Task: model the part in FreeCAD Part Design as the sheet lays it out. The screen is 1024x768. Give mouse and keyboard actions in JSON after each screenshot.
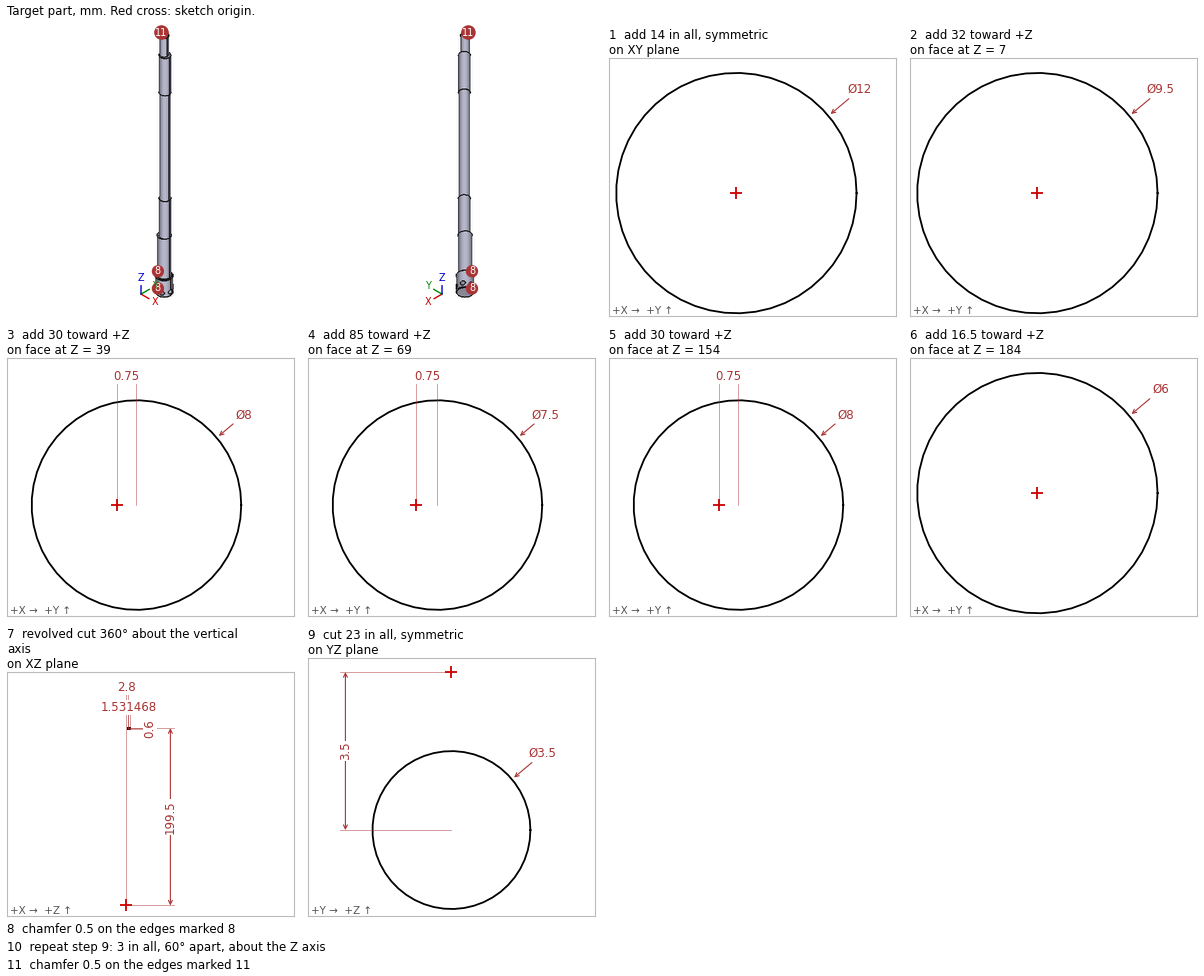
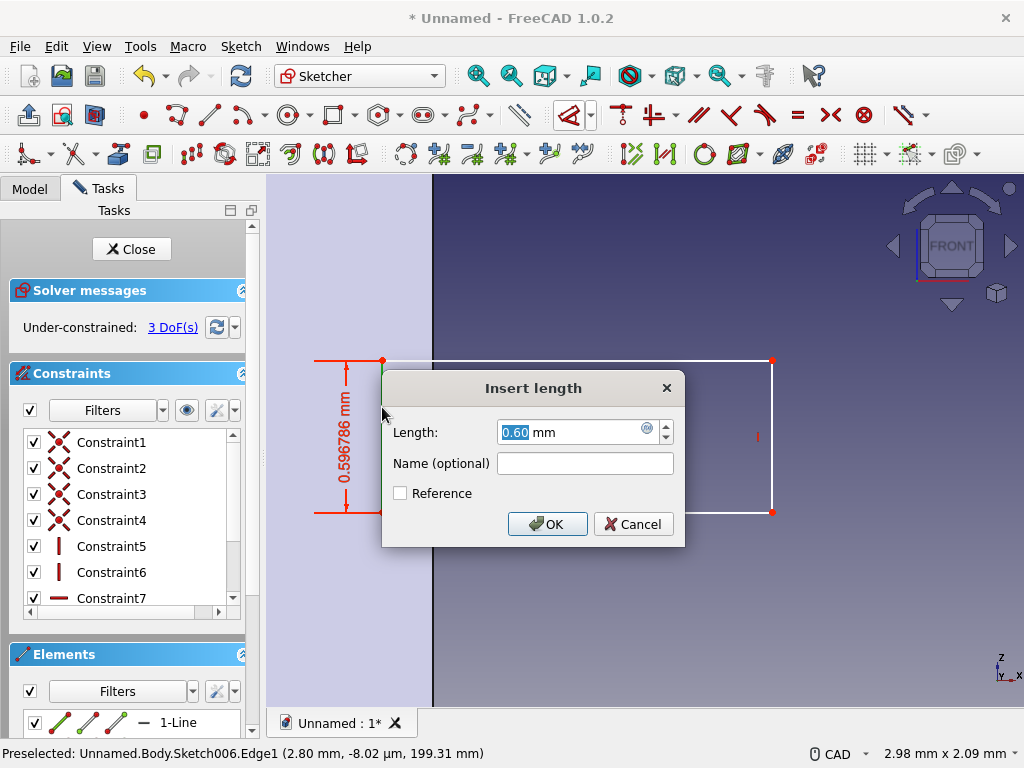
{"action": "type", "text": "0.6"}
{"action": "key", "text": "Return"}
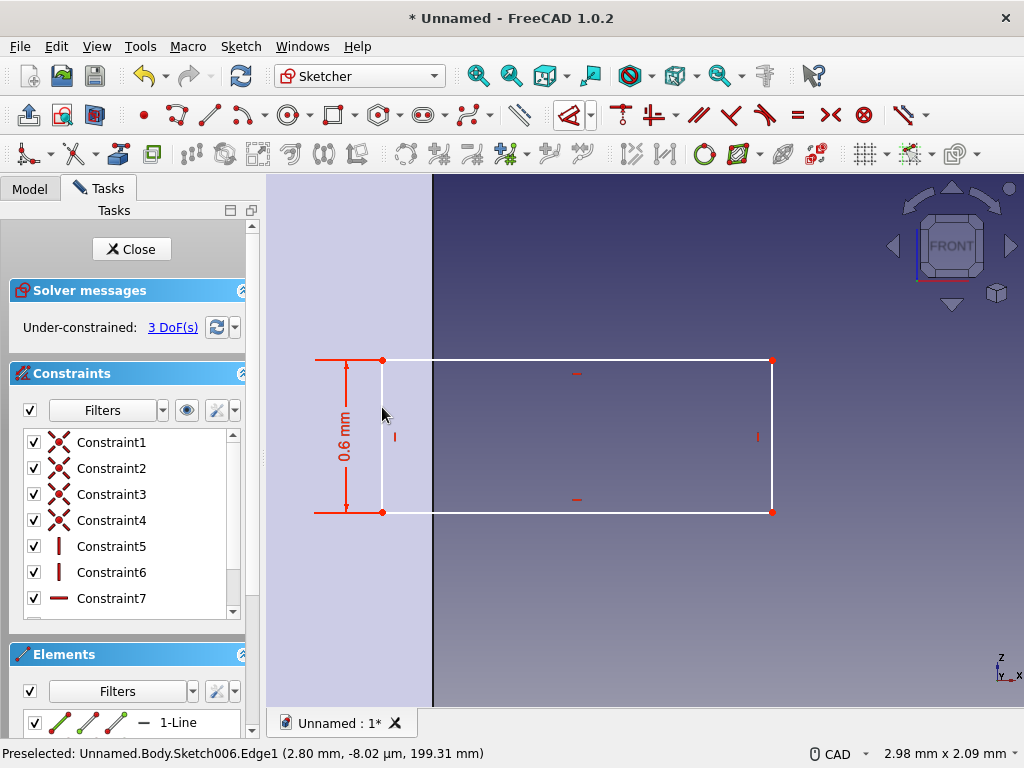
{"action": "left_click", "coordinate": [382, 360]}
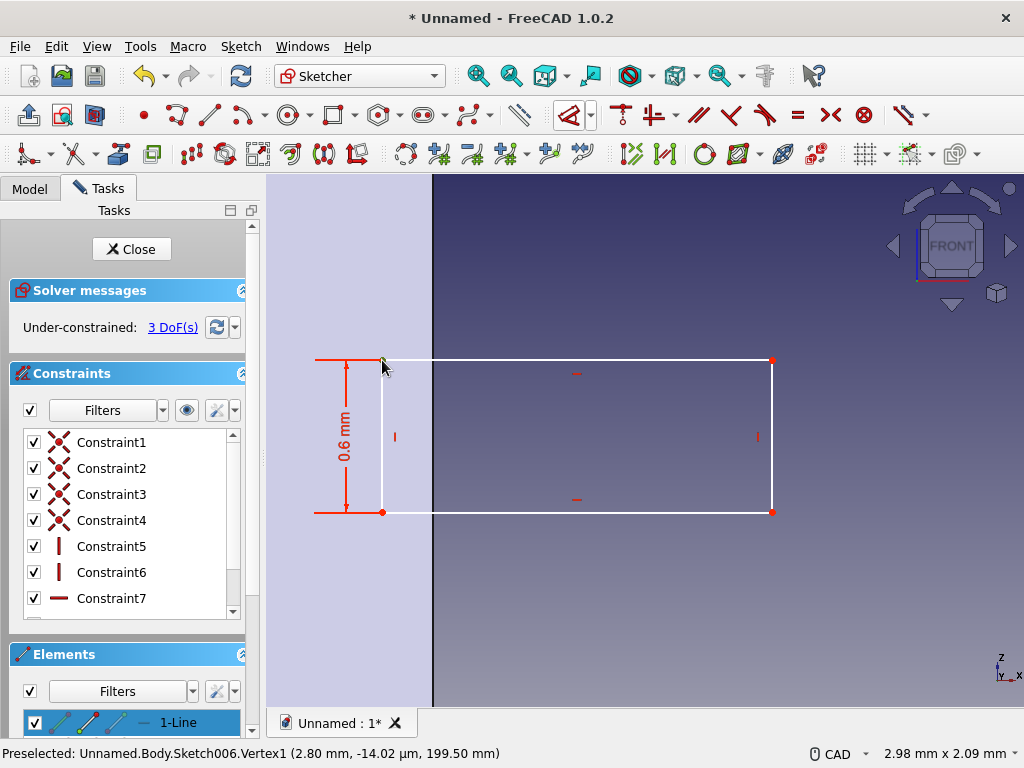
{"action": "key", "text": "l"}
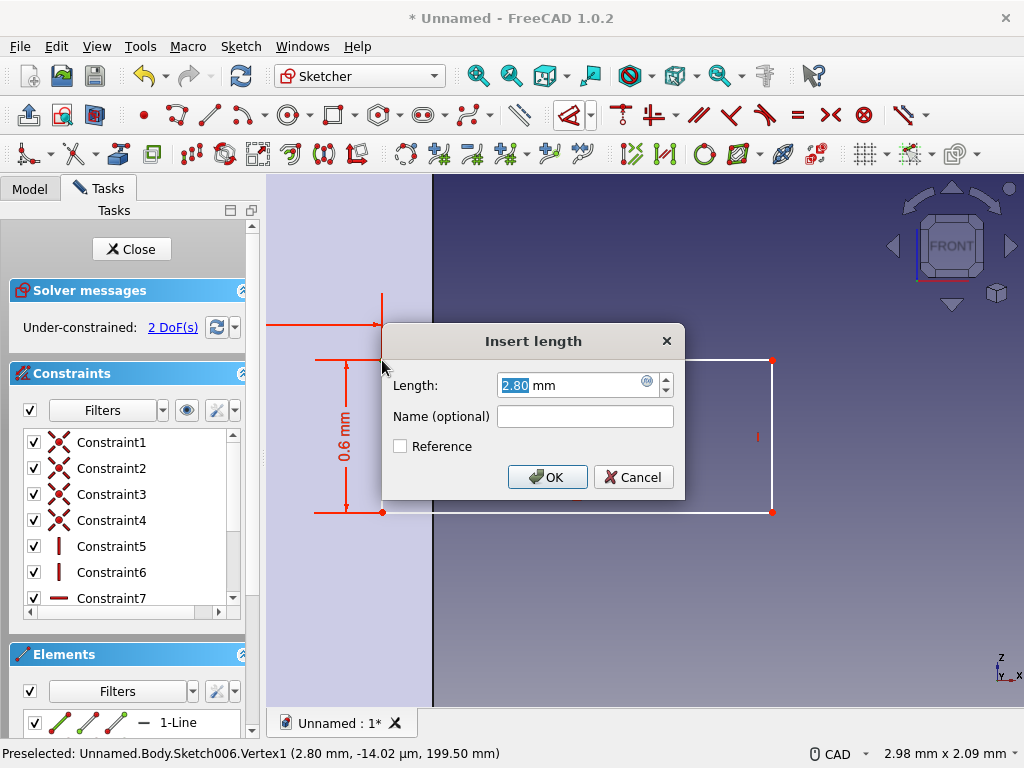
{"action": "type", "text": "2.8"}
{"action": "key", "text": "Return"}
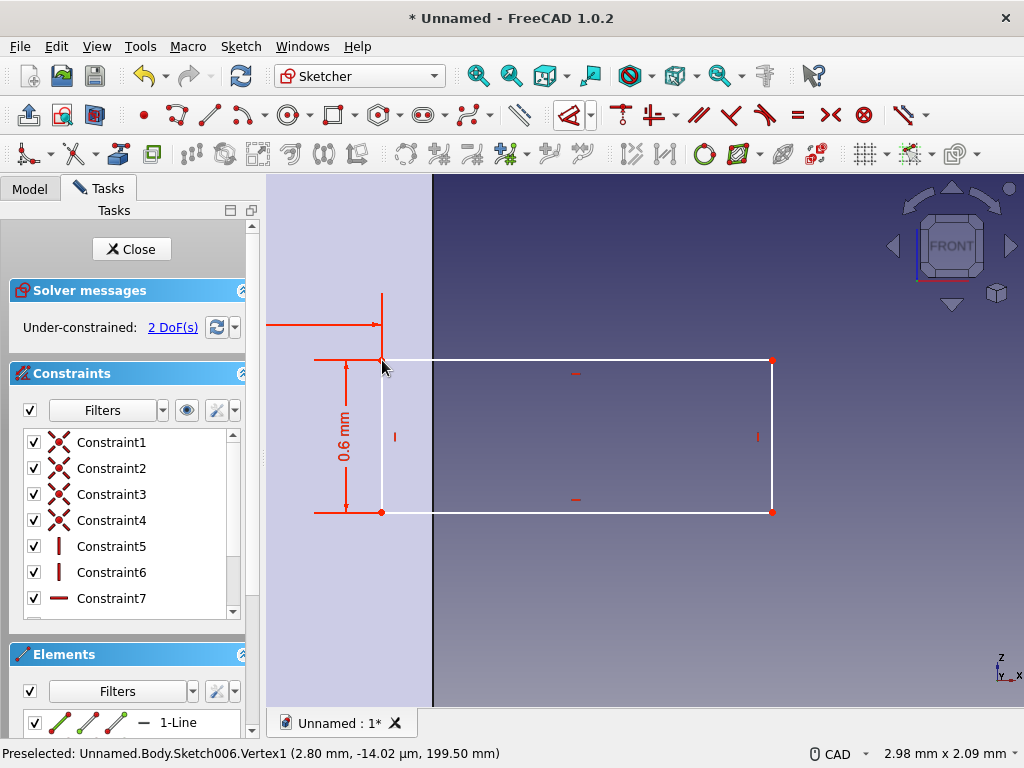
{"action": "left_click", "coordinate": [382, 360]}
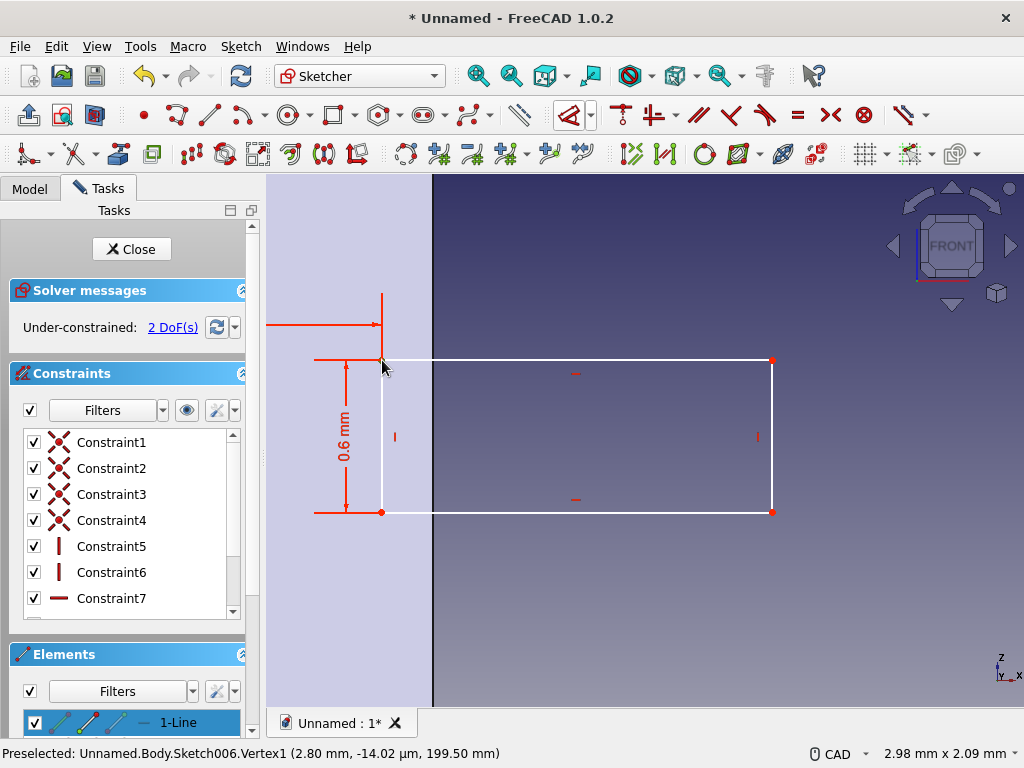
{"action": "key", "text": "i"}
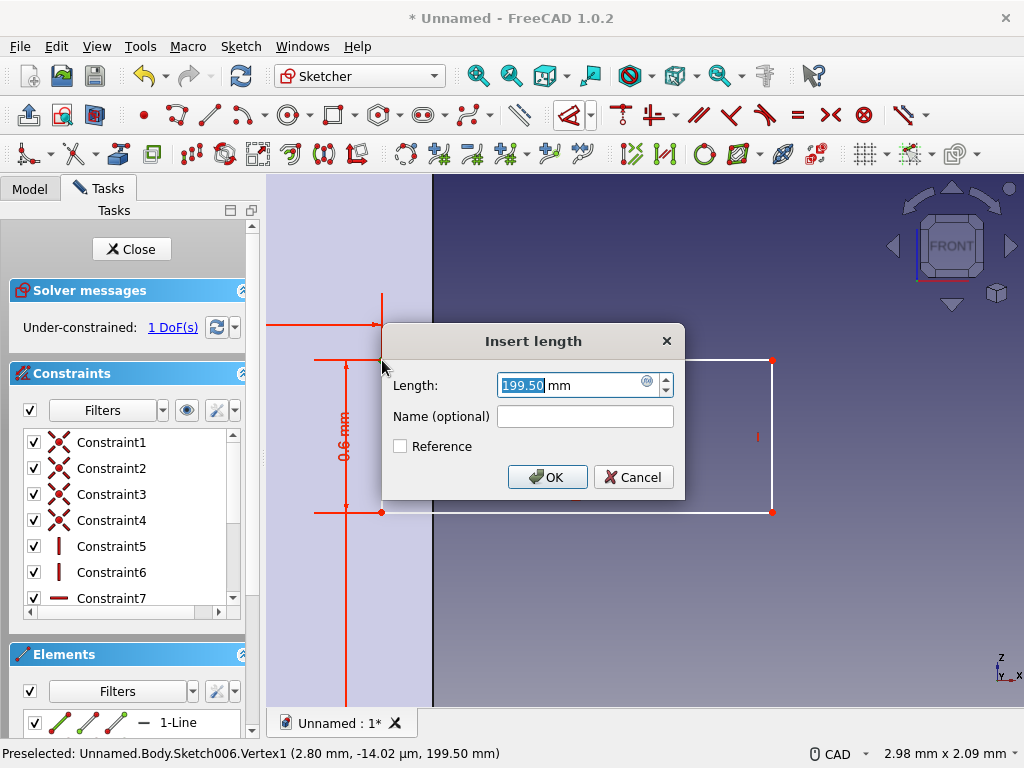
{"action": "type", "text": "199.5"}
{"action": "key", "text": "Return"}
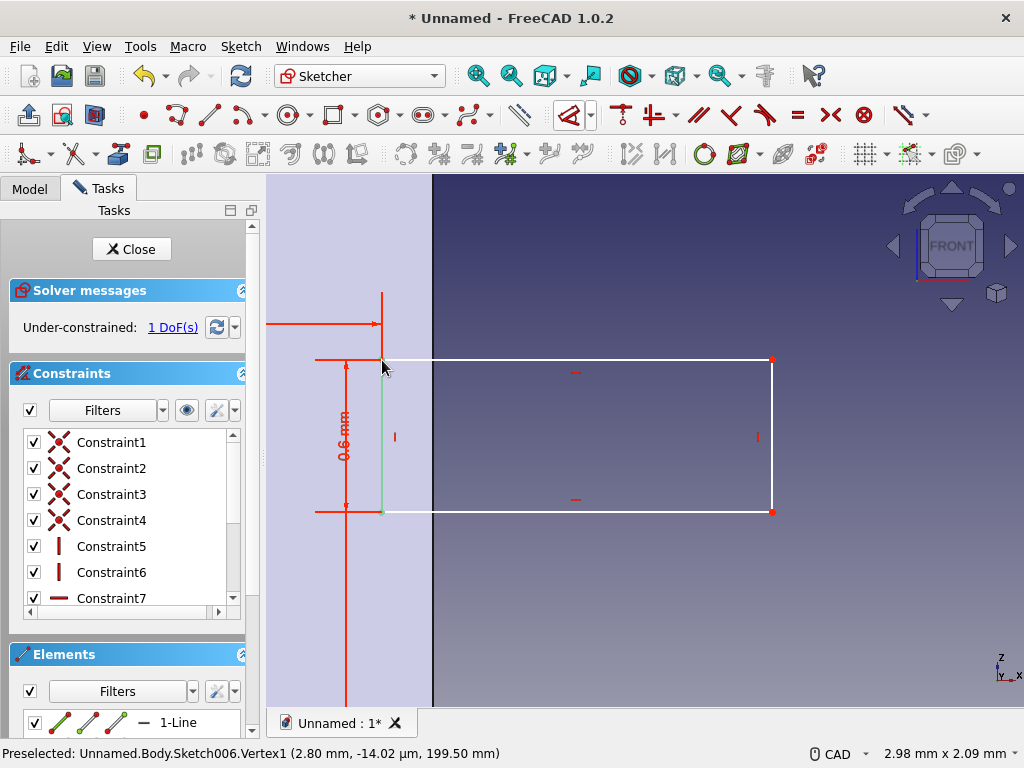
{"action": "left_click", "coordinate": [499, 512]}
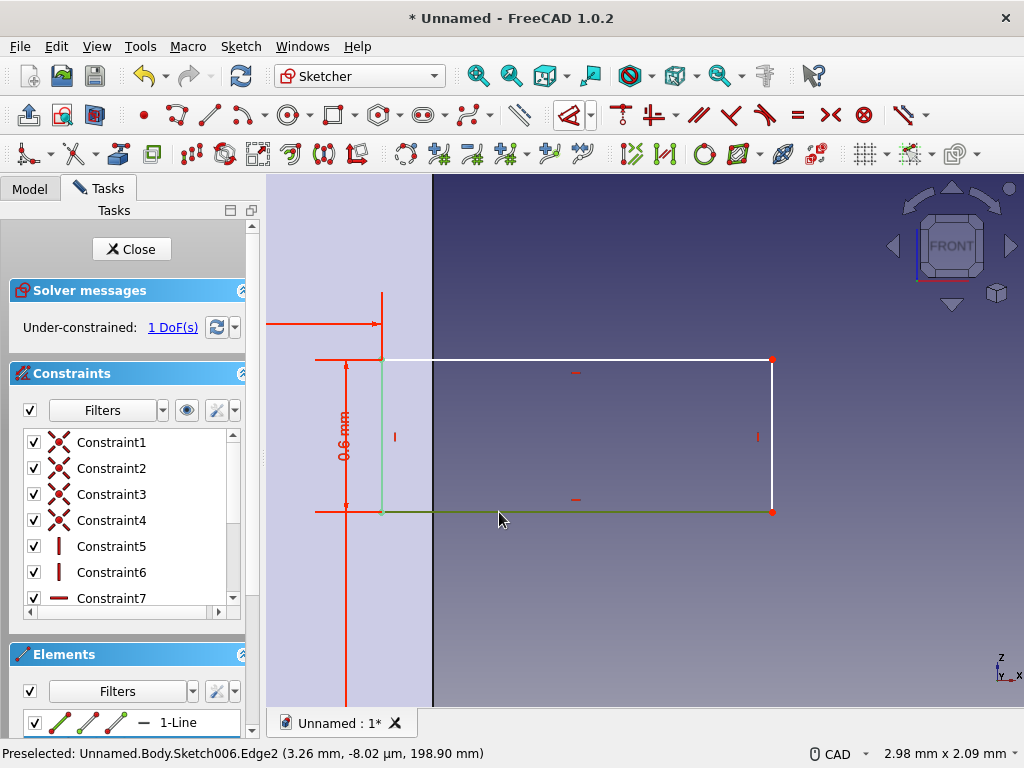
{"action": "key", "text": "l"}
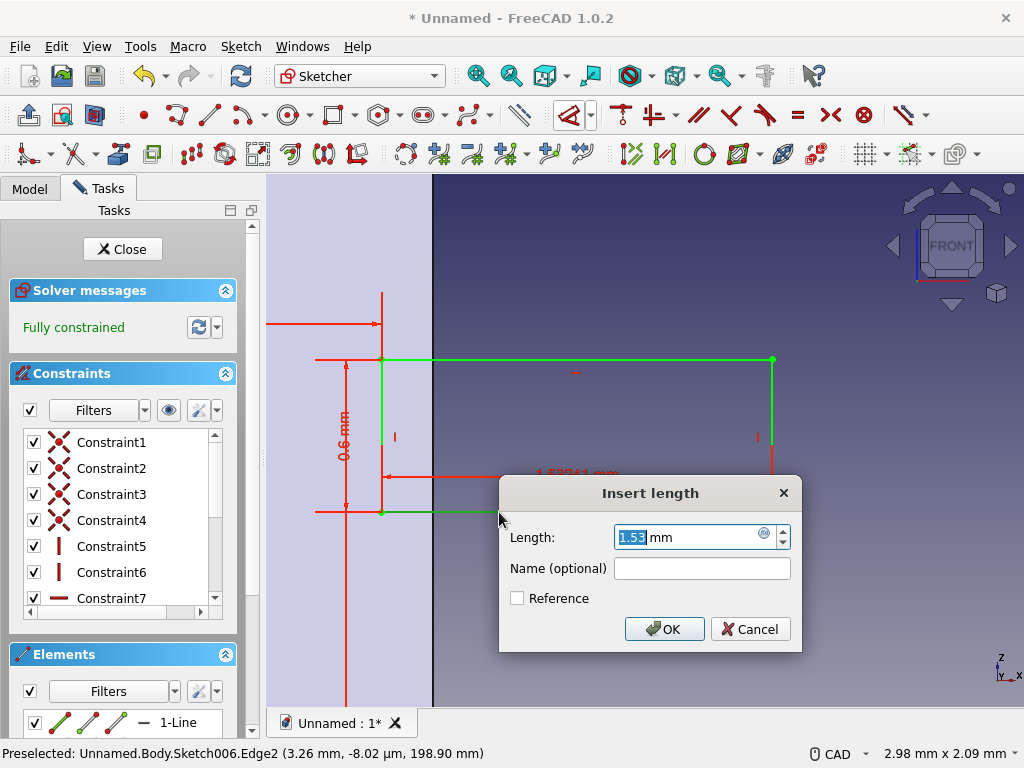
{"action": "type", "text": "1.531468"}
{"action": "key", "text": "Return"}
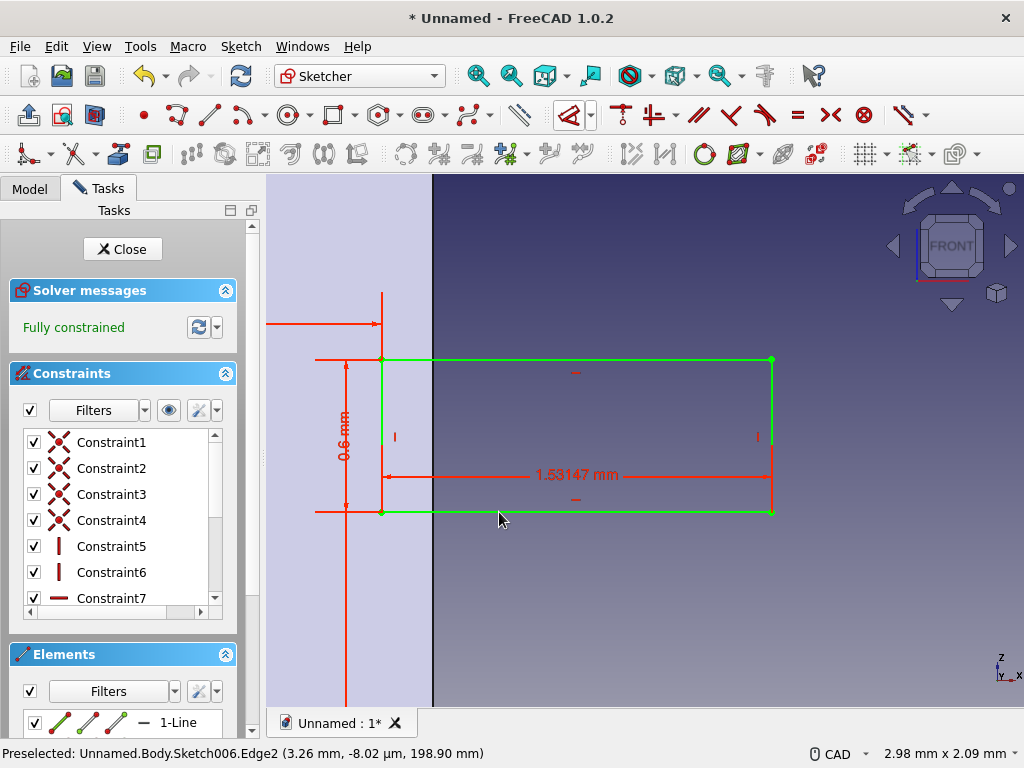
{"action": "left_click", "coordinate": [123, 249]}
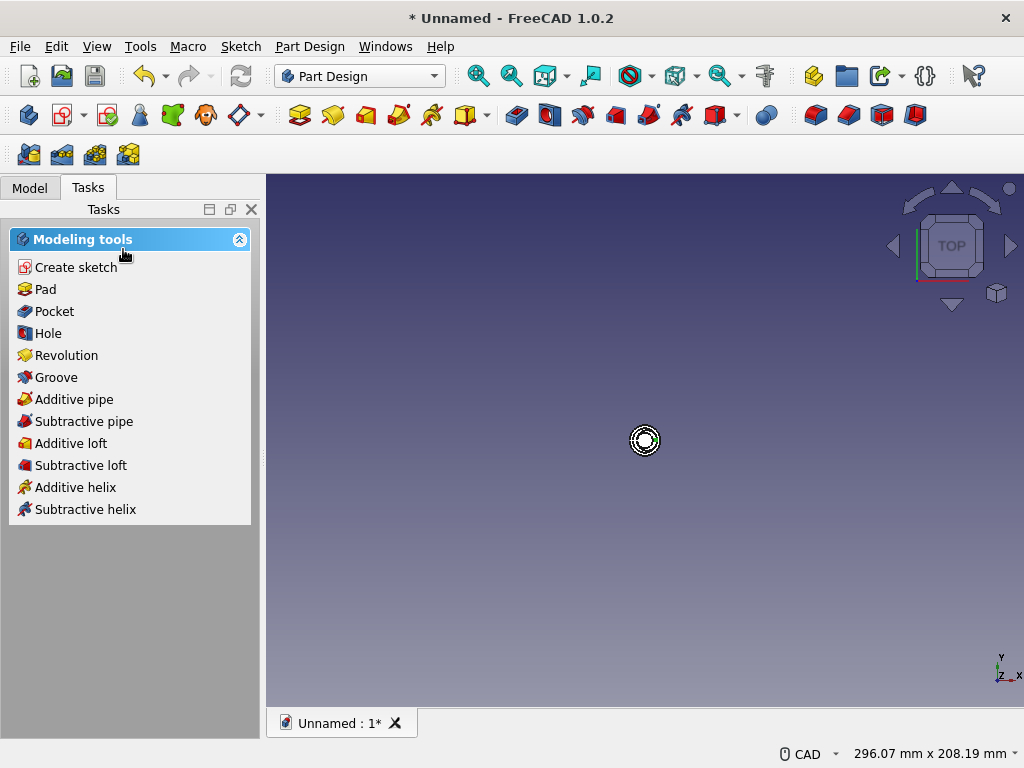
{"action": "left_click", "coordinate": [583, 116]}